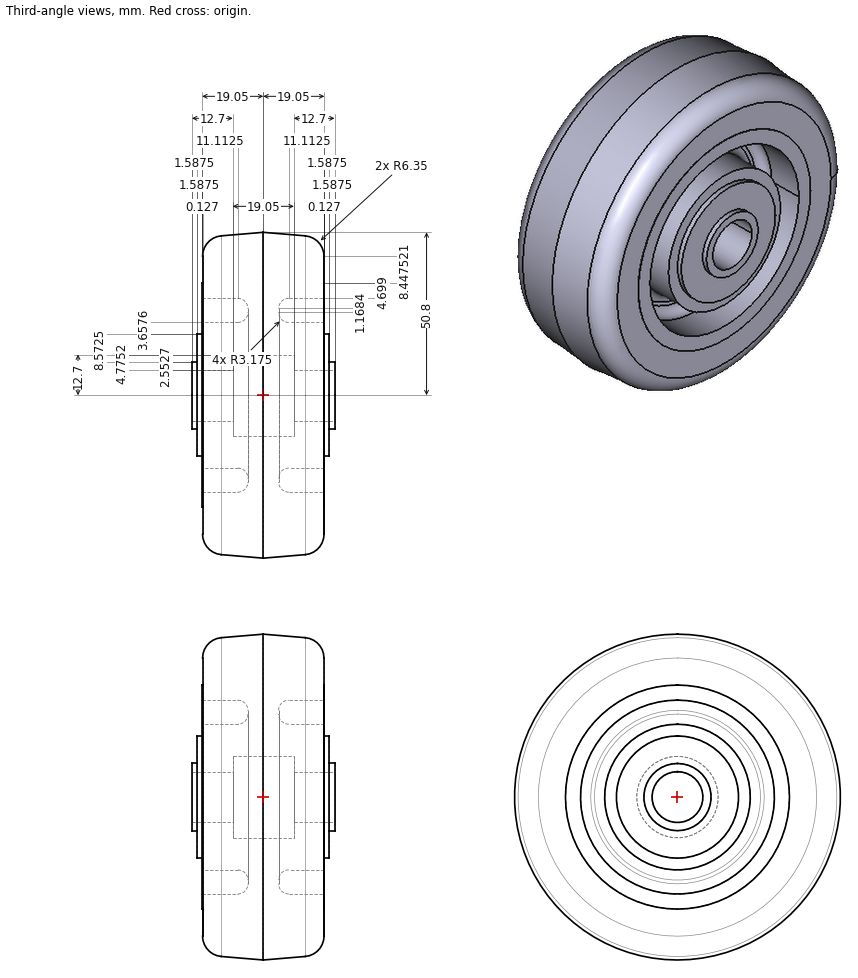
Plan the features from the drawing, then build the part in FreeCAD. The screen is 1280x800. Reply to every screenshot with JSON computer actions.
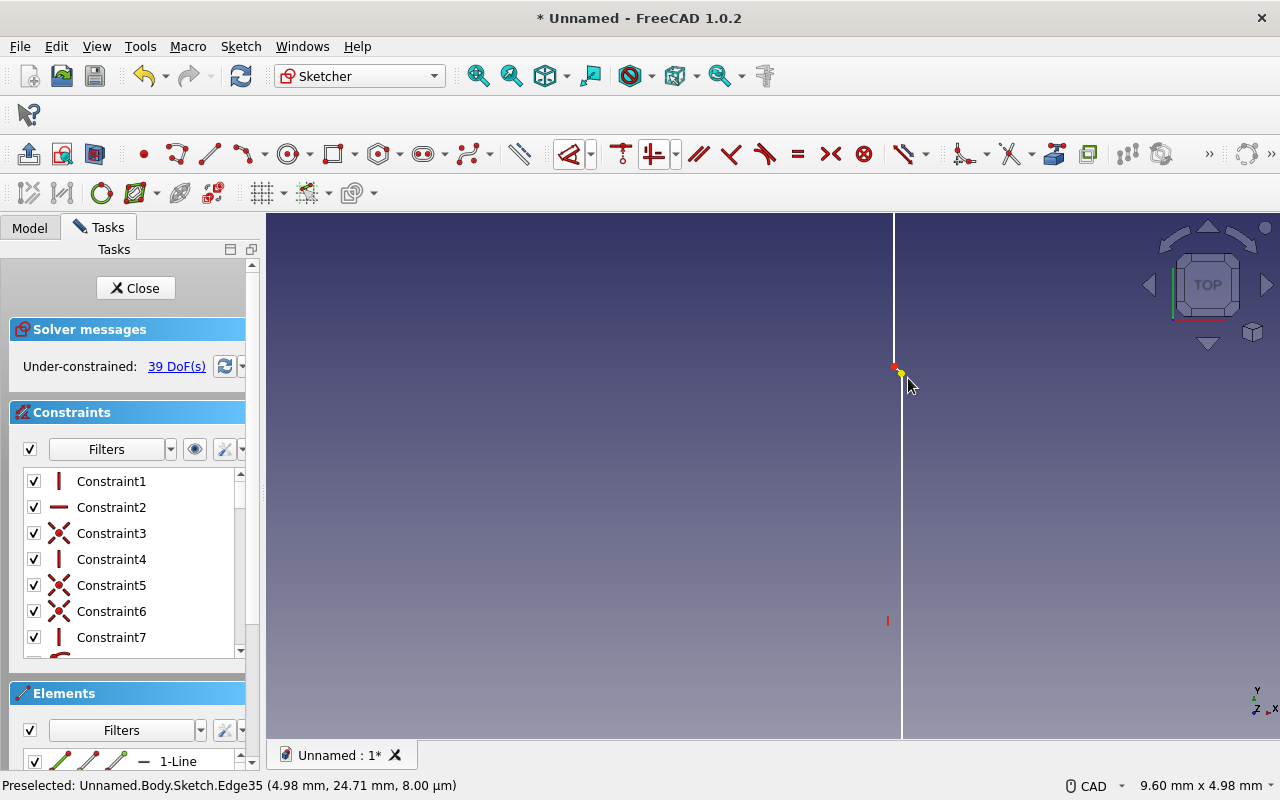
{"action": "scroll", "coordinate": [898, 370], "scroll_direction": "up", "scroll_amount": 4}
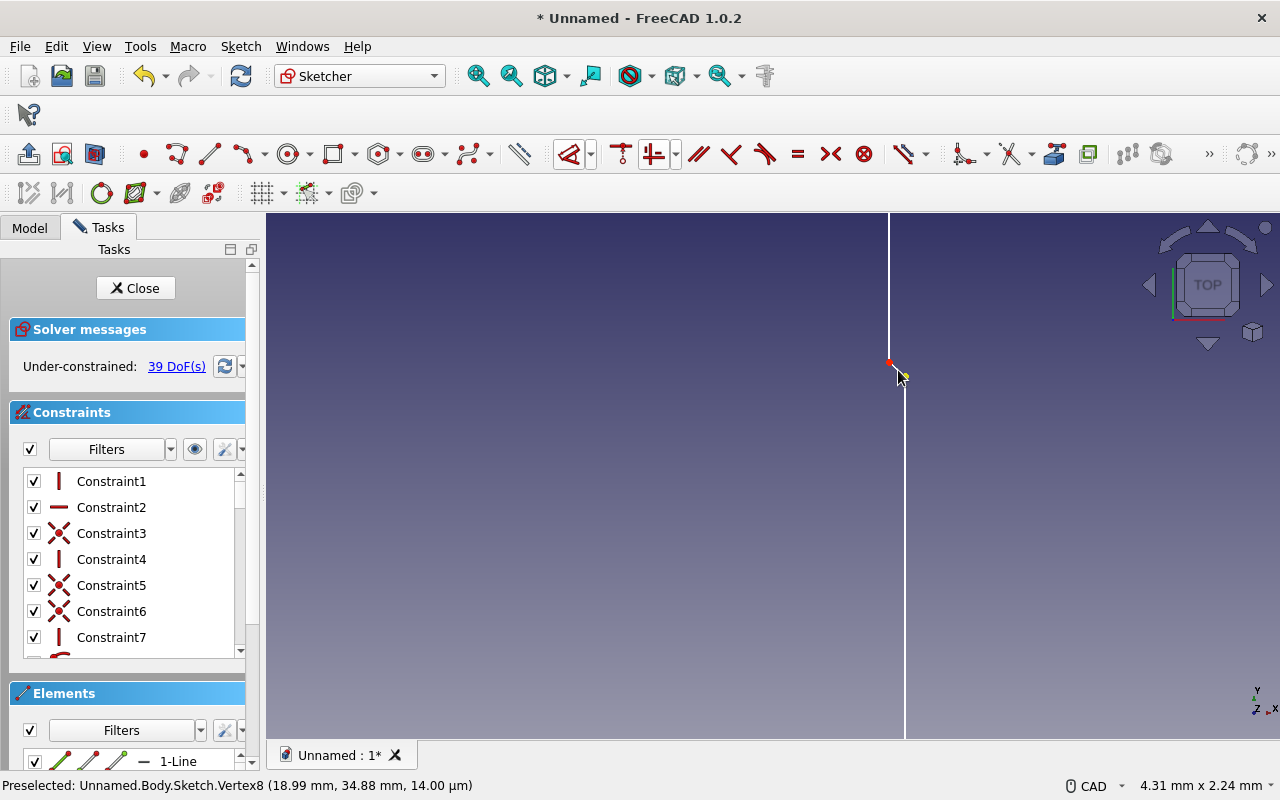
{"action": "left_click", "coordinate": [897, 370]}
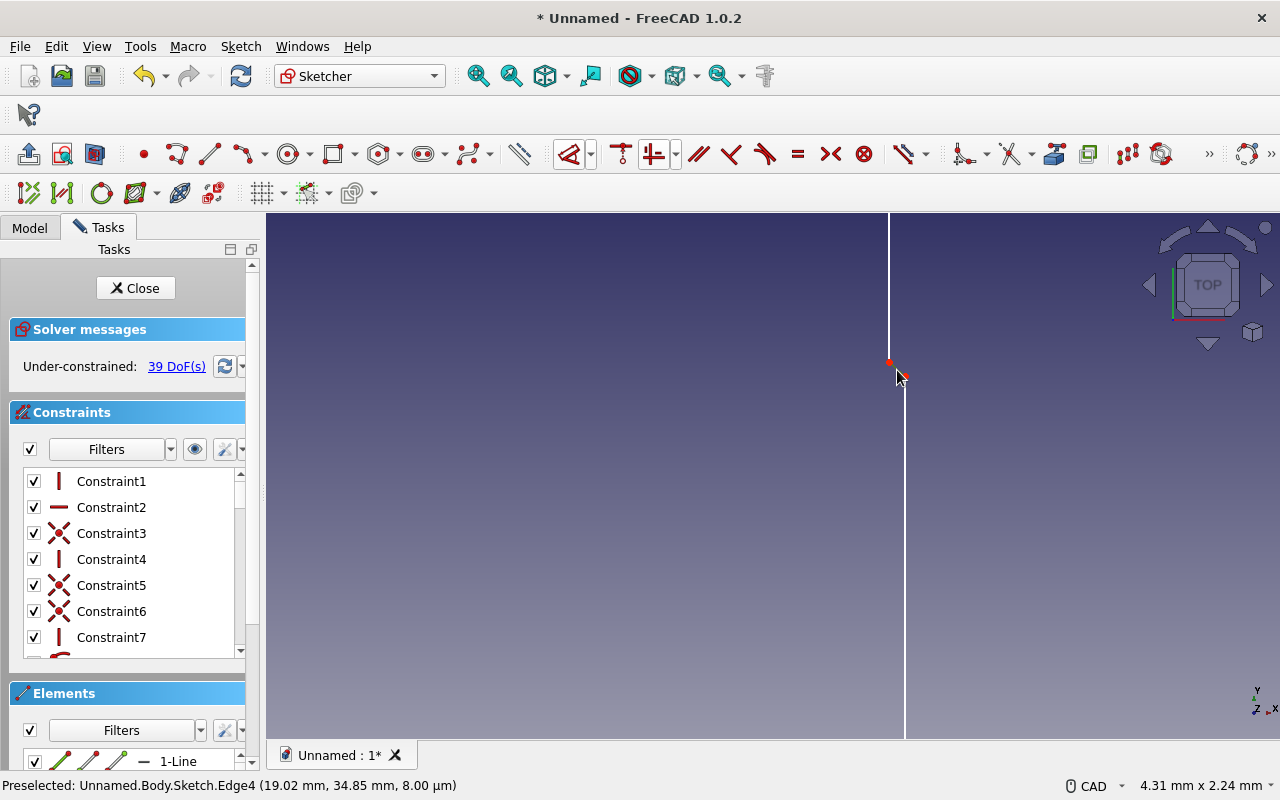
{"action": "left_click", "coordinate": [676, 154]}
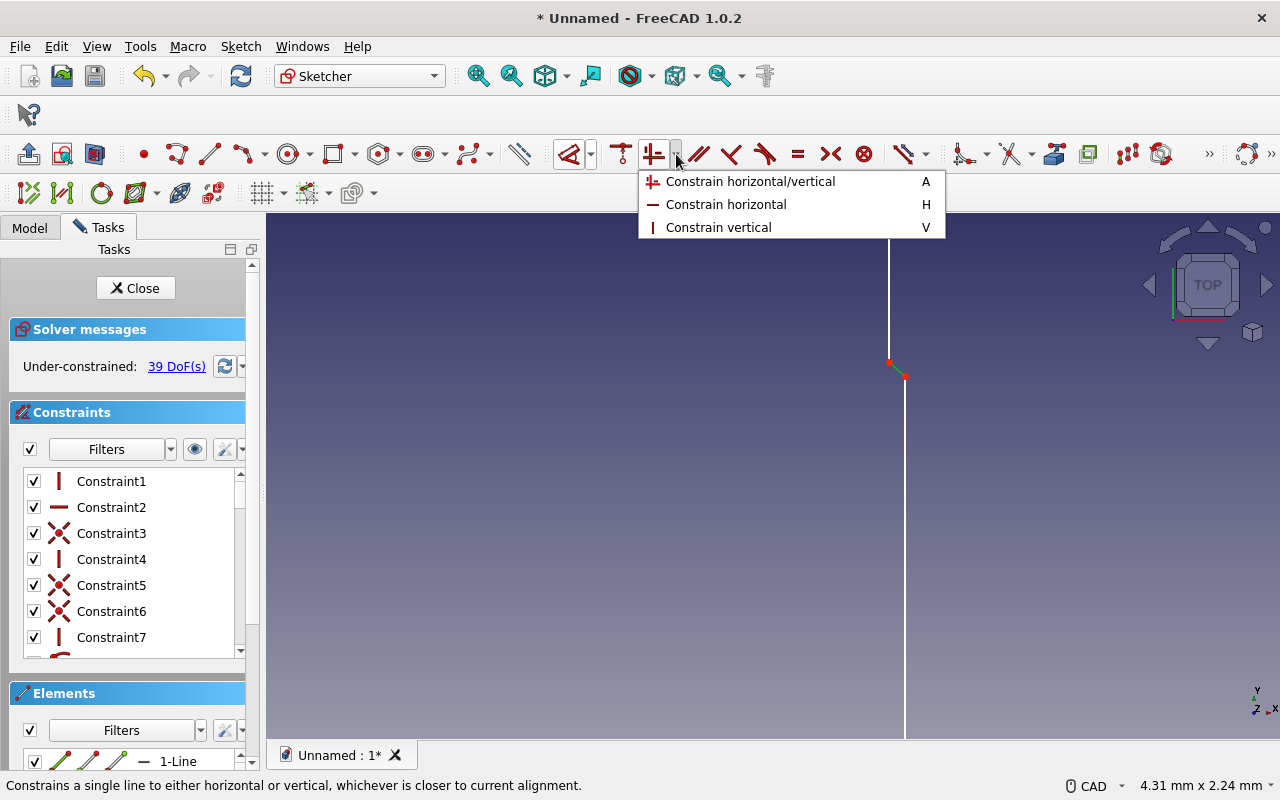
{"action": "left_click", "coordinate": [792, 204]}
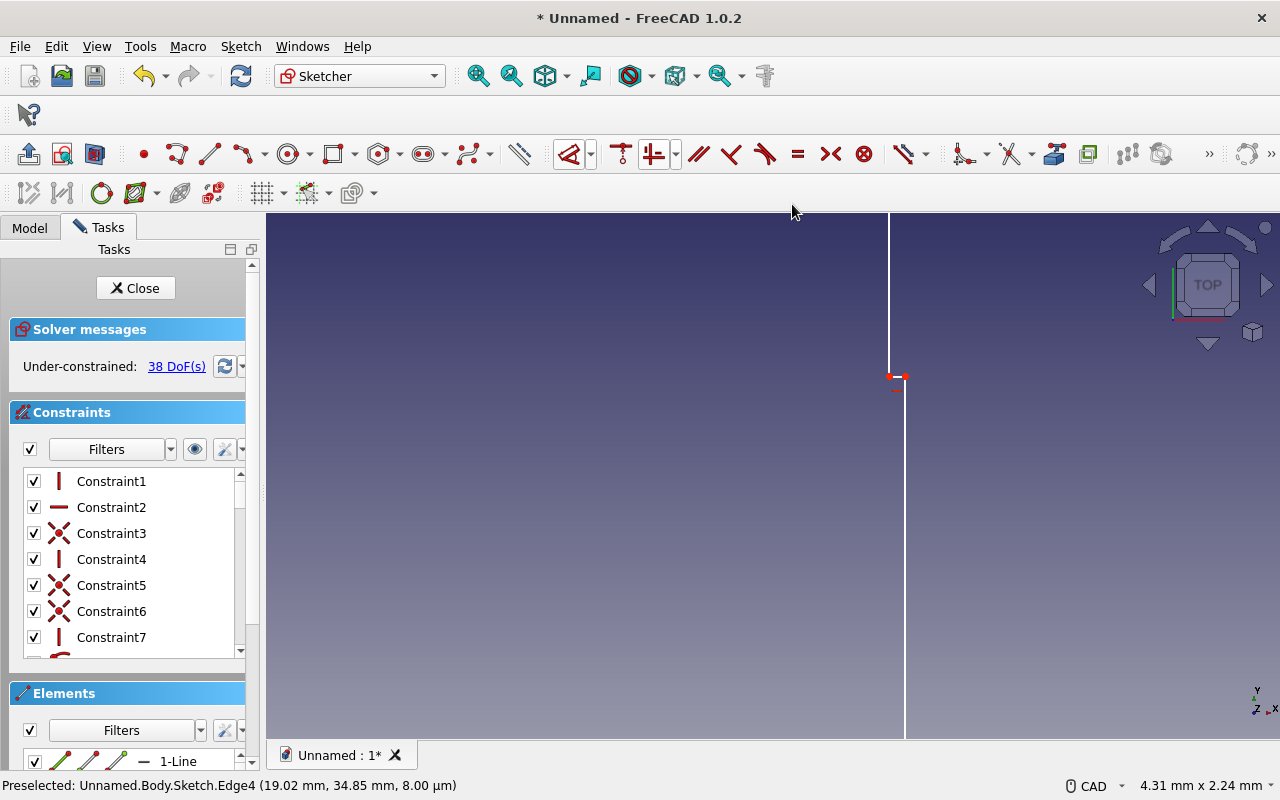
{"action": "scroll", "coordinate": [852, 403], "scroll_direction": "down", "scroll_amount": 17}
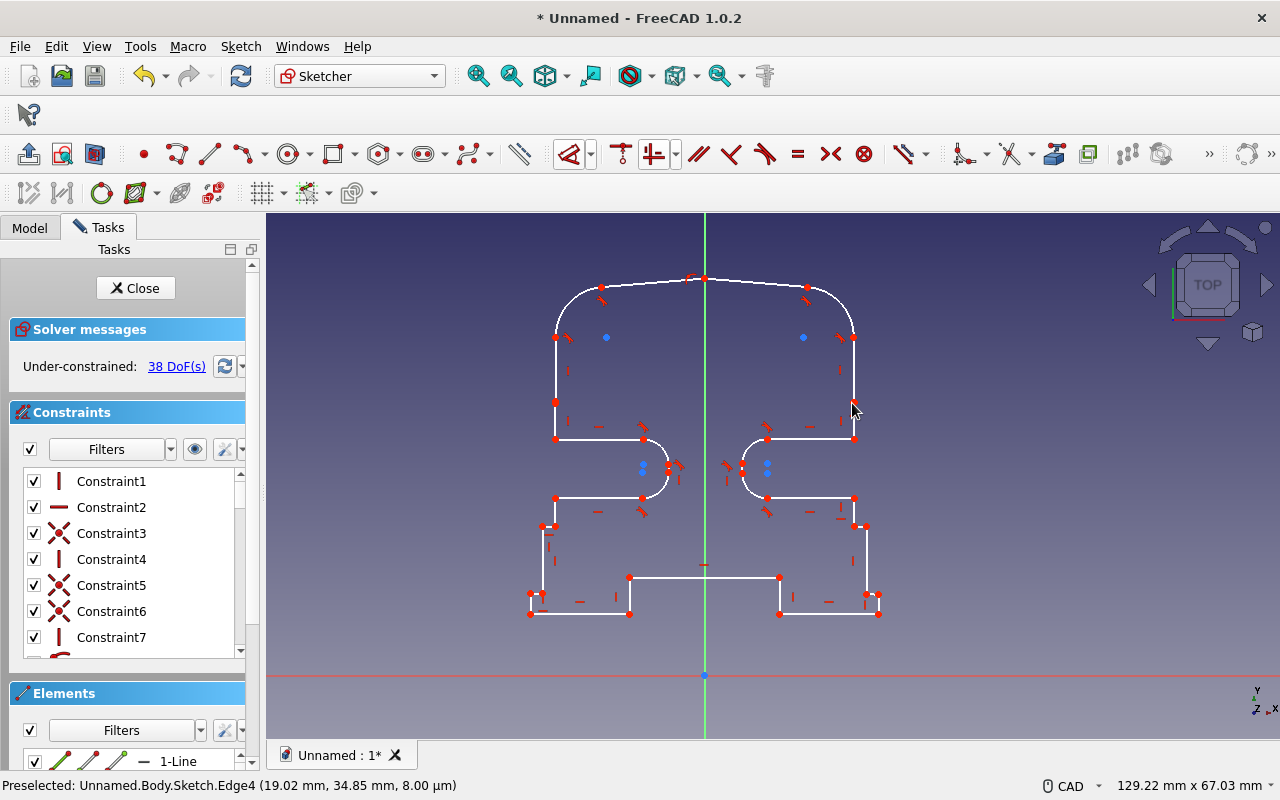
{"action": "scroll", "coordinate": [556, 403], "scroll_direction": "up", "scroll_amount": 13}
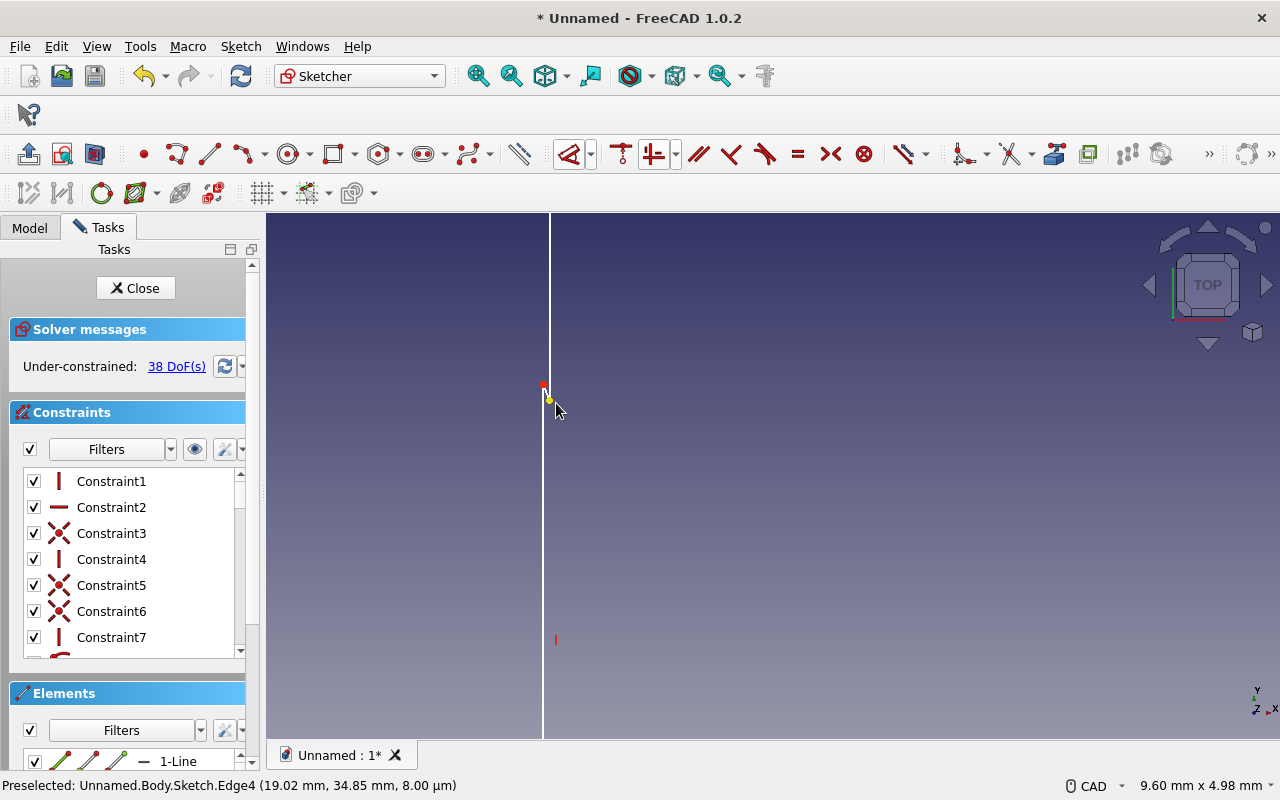
{"action": "scroll", "coordinate": [546, 392], "scroll_direction": "up", "scroll_amount": 4}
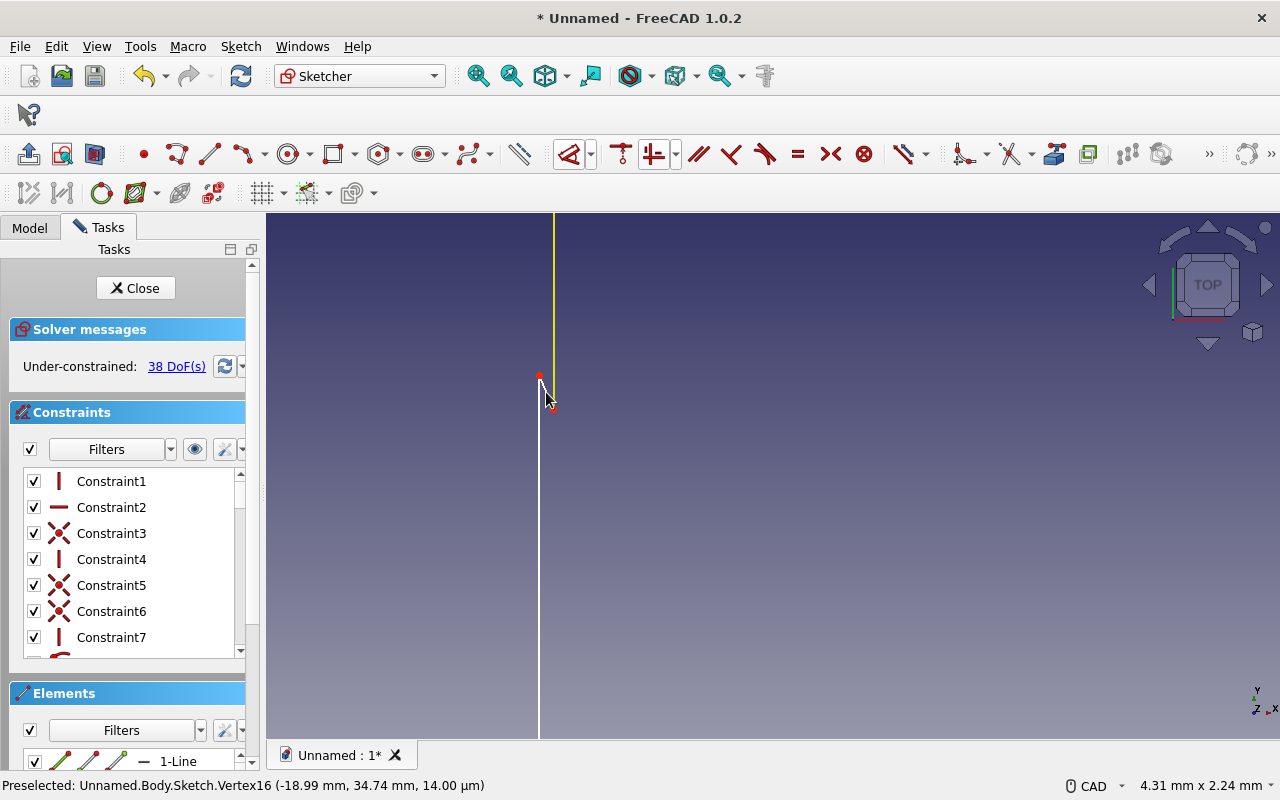
{"action": "left_click", "coordinate": [546, 392]}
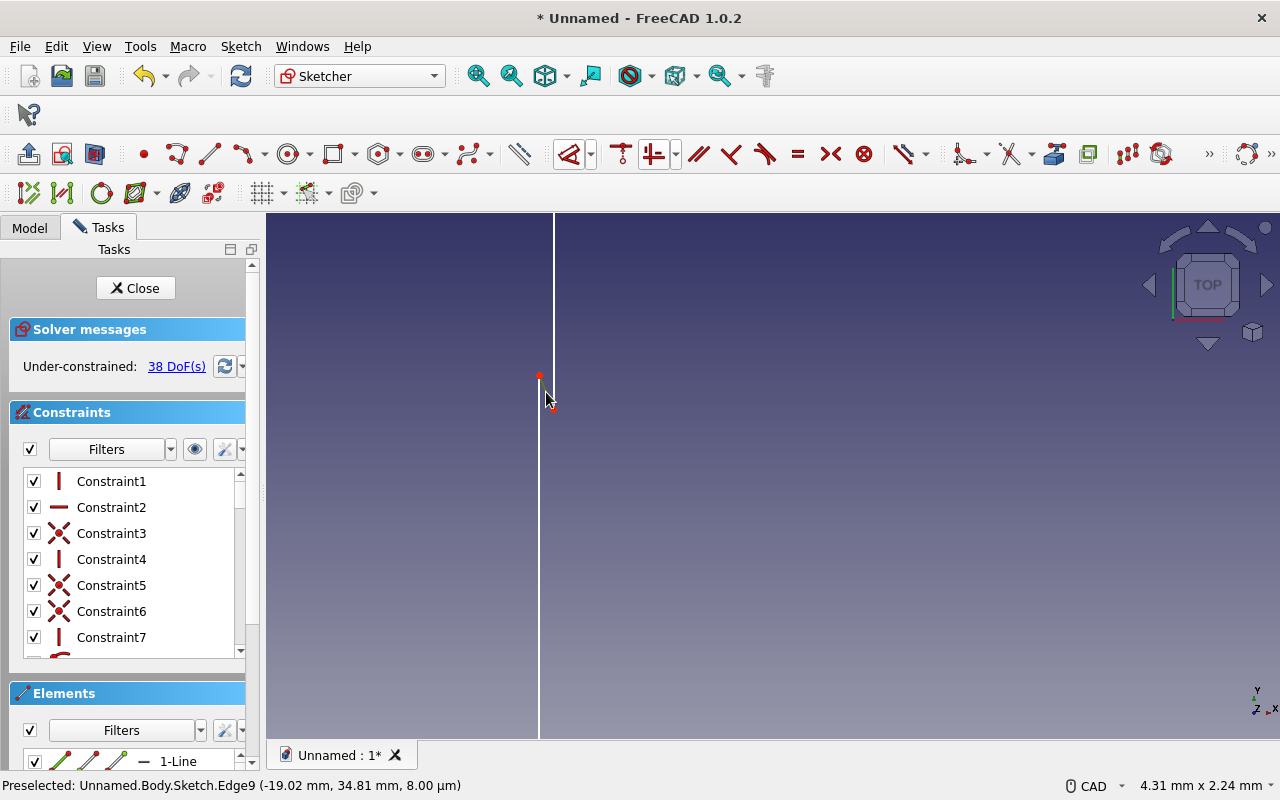
{"action": "left_click", "coordinate": [676, 154]}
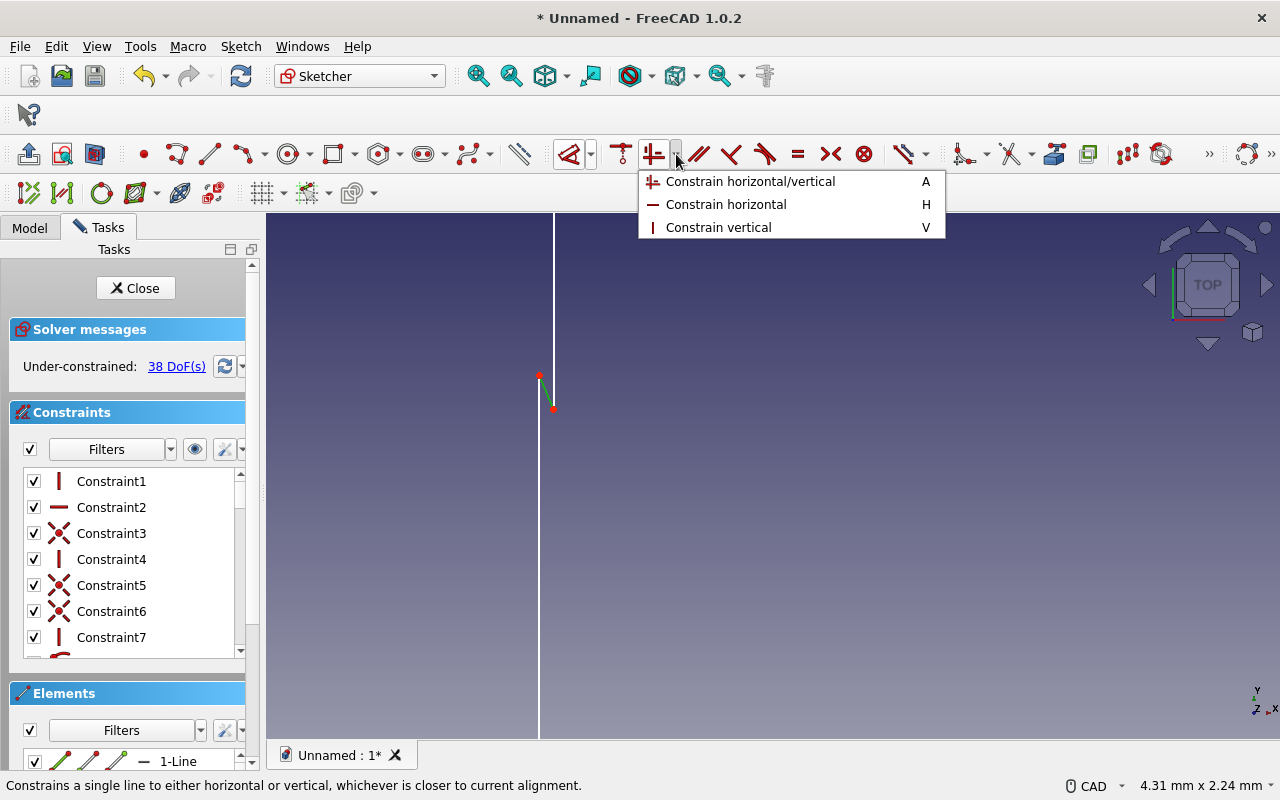
{"action": "left_click", "coordinate": [792, 204]}